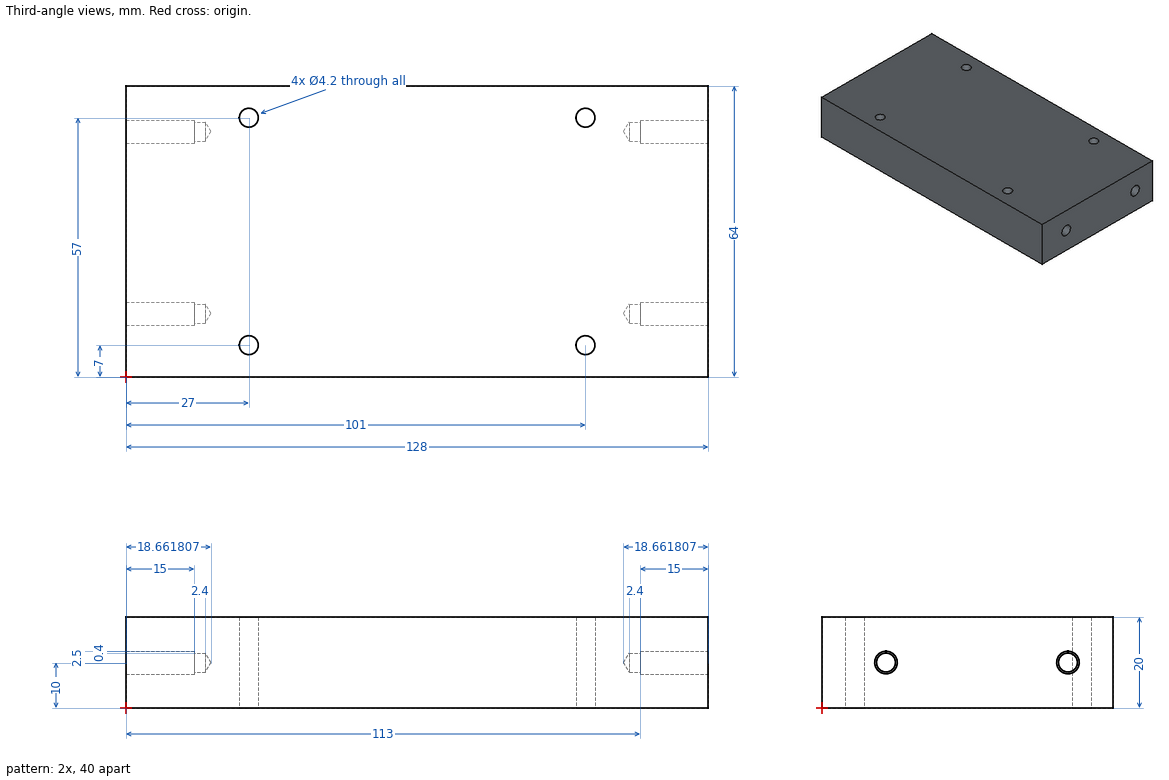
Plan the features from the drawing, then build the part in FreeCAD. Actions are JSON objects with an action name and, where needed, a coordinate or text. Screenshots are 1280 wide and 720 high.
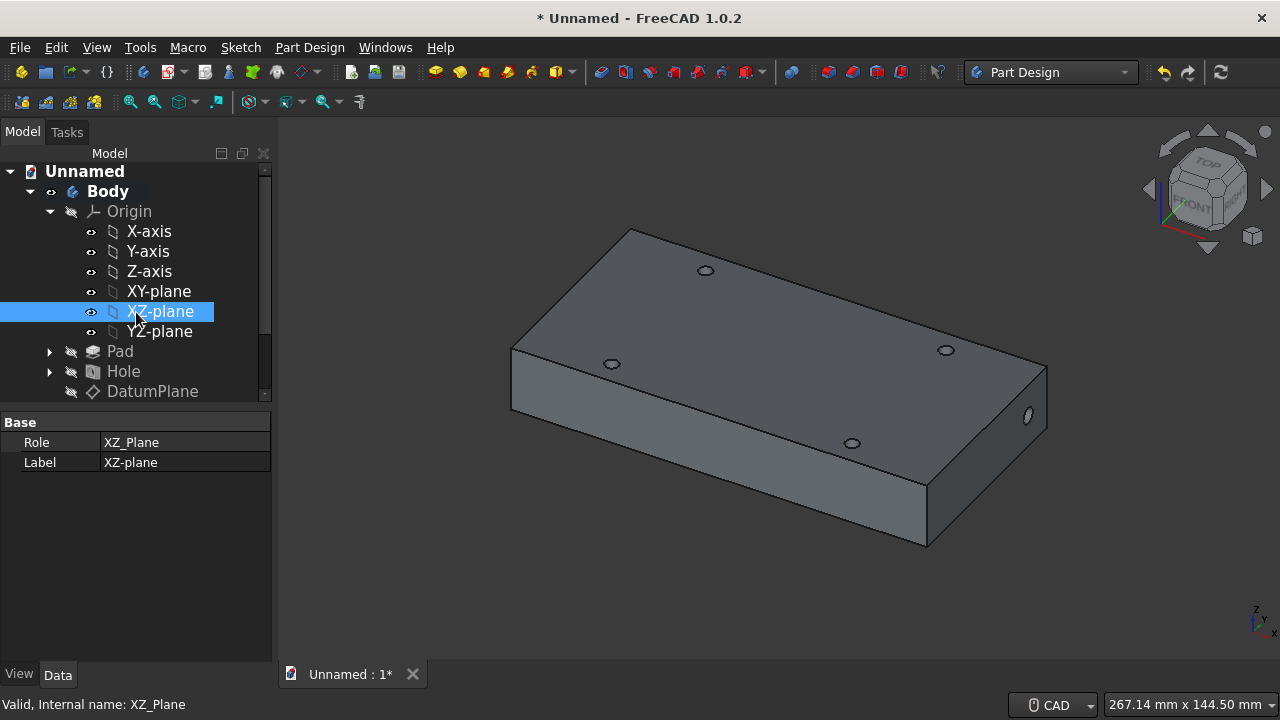
{"action": "left_click", "coordinate": [302, 72]}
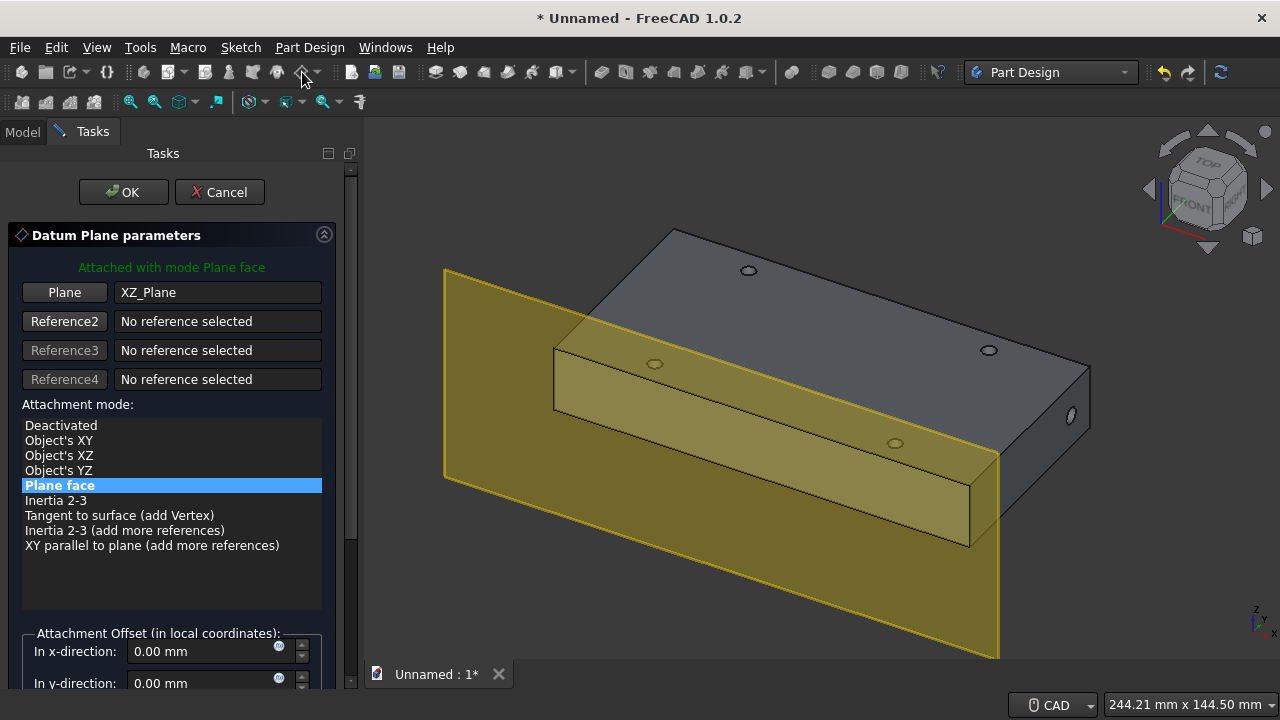
{"action": "scroll", "coordinate": [351, 426], "scroll_direction": "down", "scroll_amount": 2}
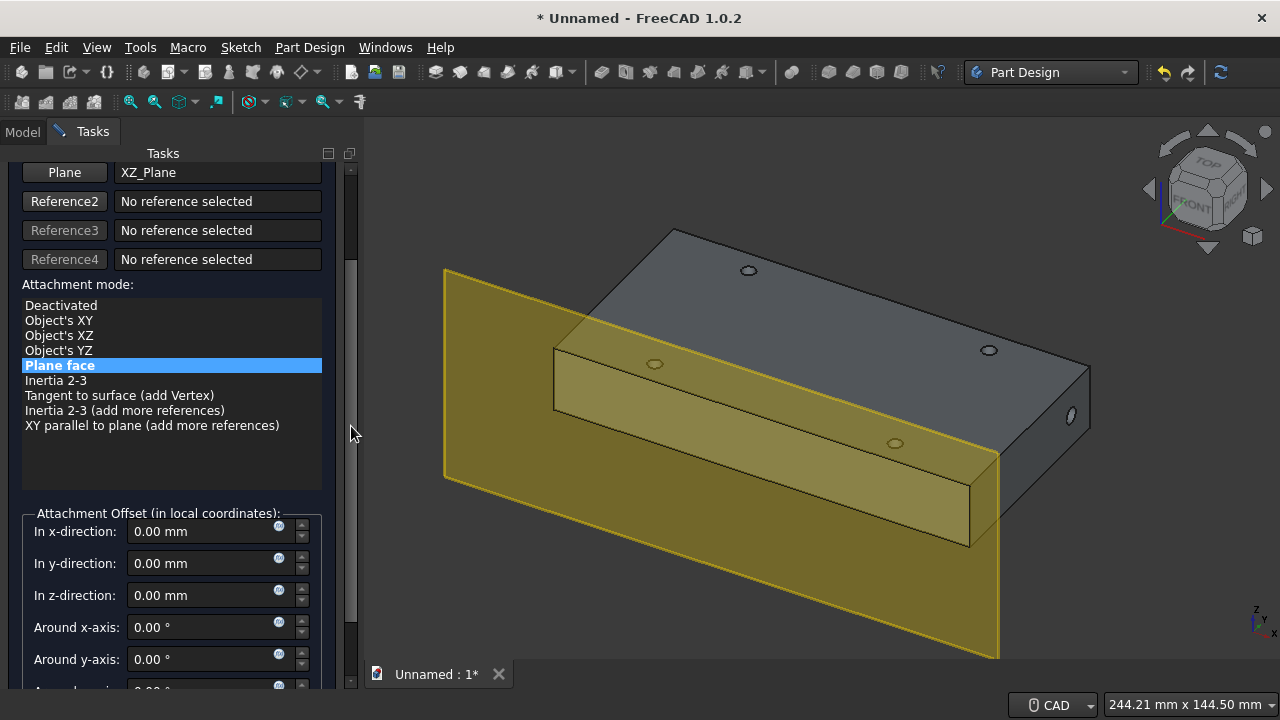
{"action": "triple_click", "coordinate": [210, 595]}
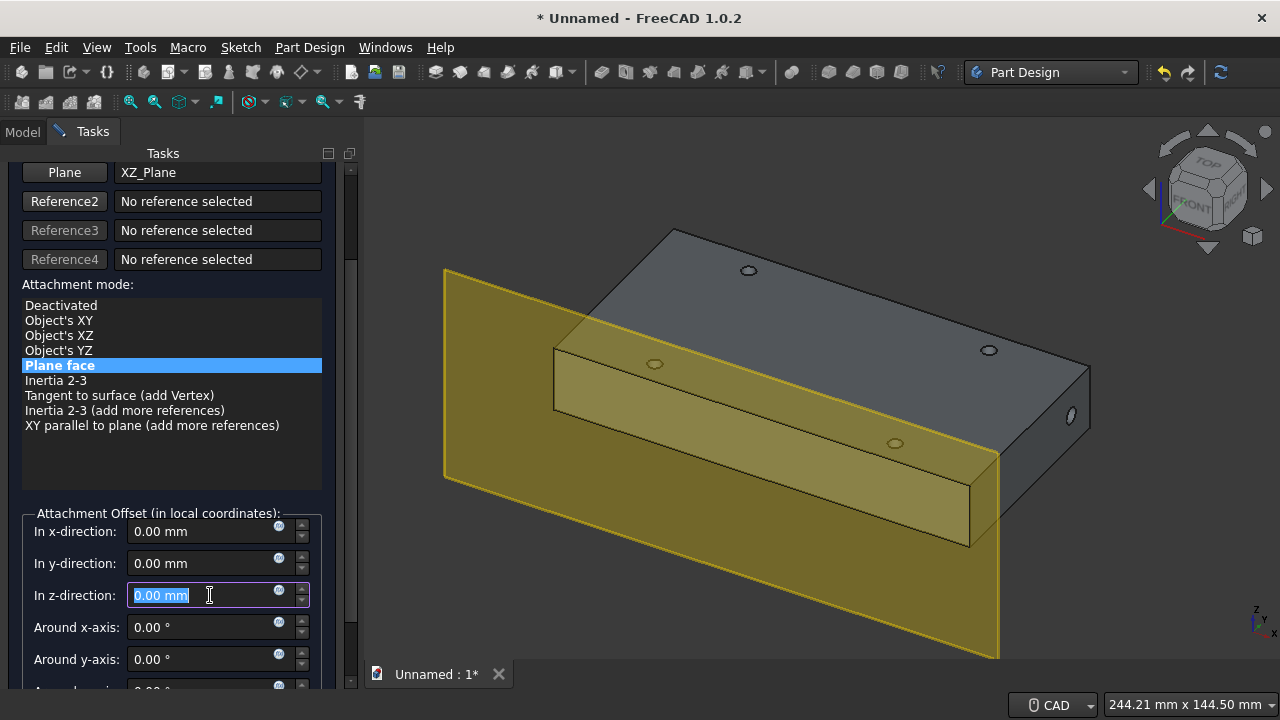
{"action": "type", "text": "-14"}
{"action": "key", "text": "Tab"}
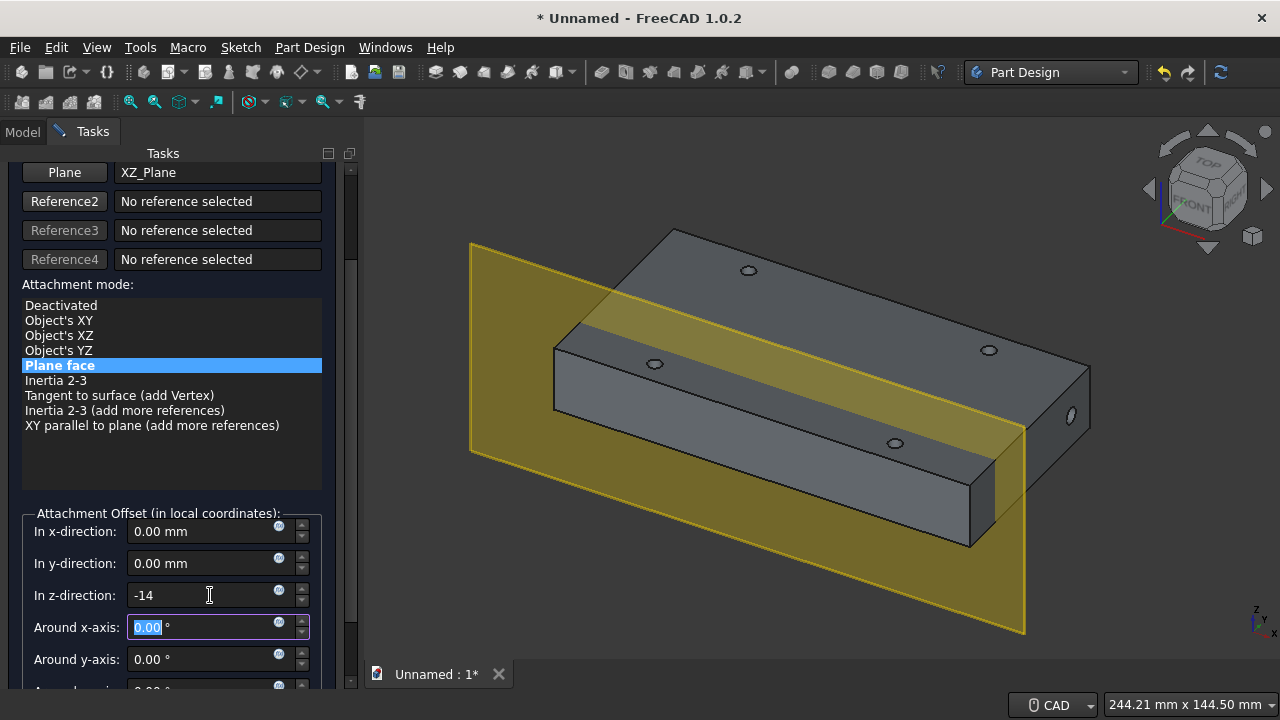
{"action": "scroll", "coordinate": [351, 426], "scroll_direction": "up", "scroll_amount": 3}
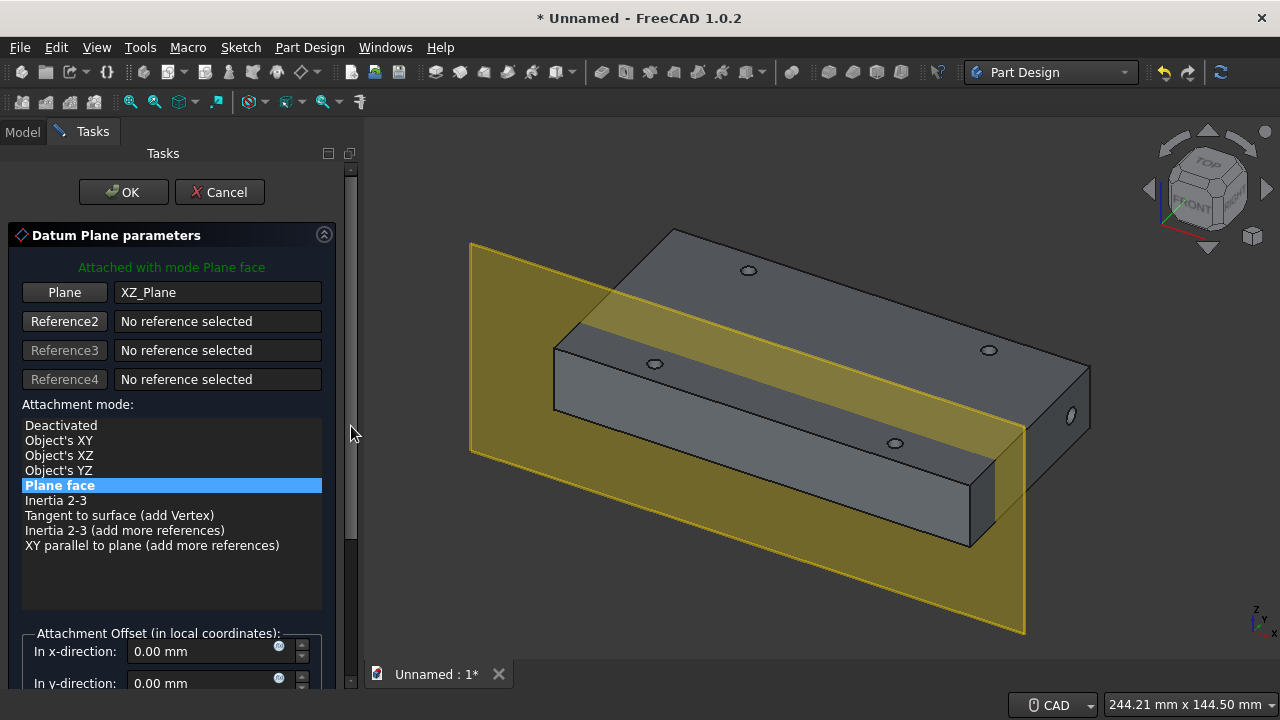
{"action": "left_click", "coordinate": [124, 192]}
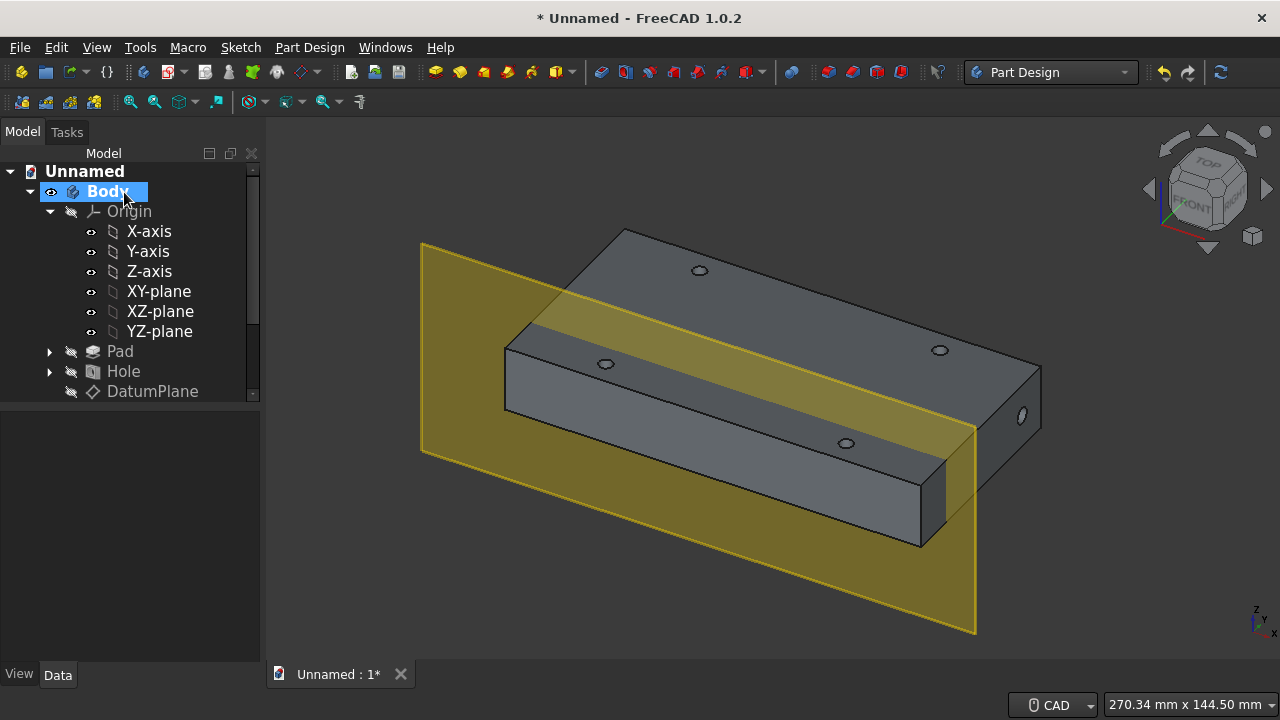
{"action": "scroll", "coordinate": [100, 287], "scroll_direction": "down", "scroll_amount": 3}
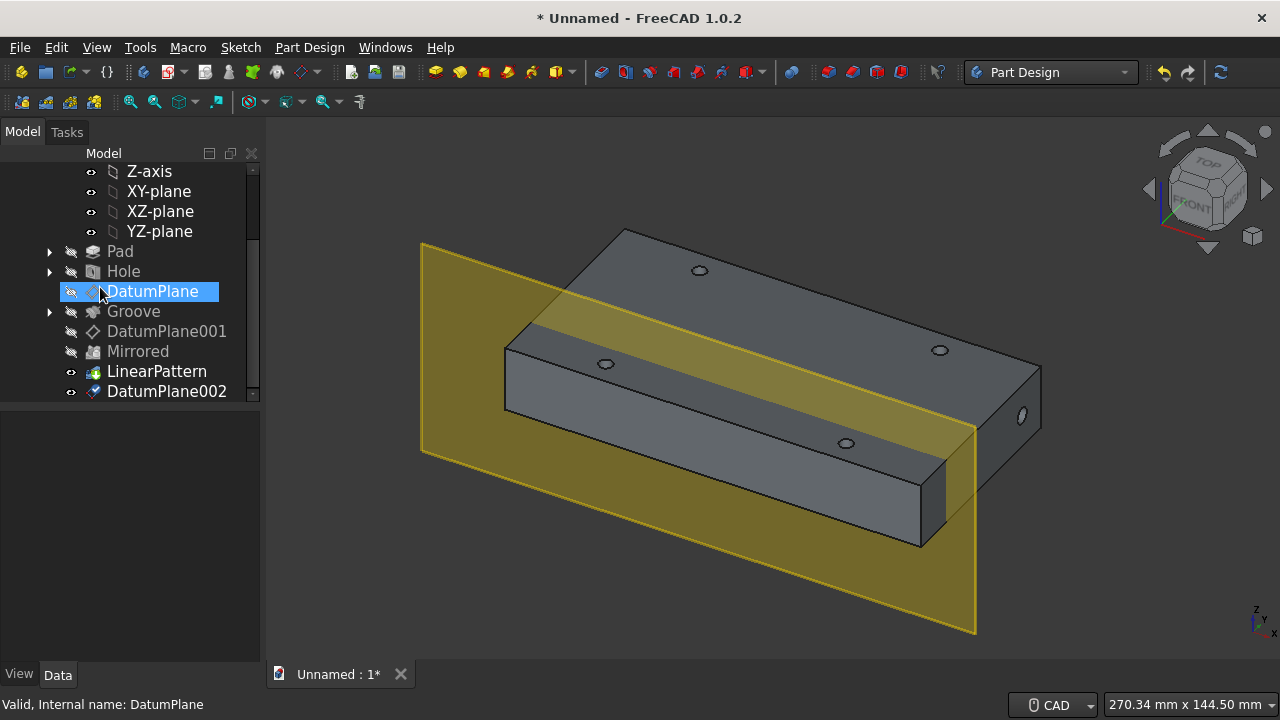
{"action": "left_click", "coordinate": [116, 392]}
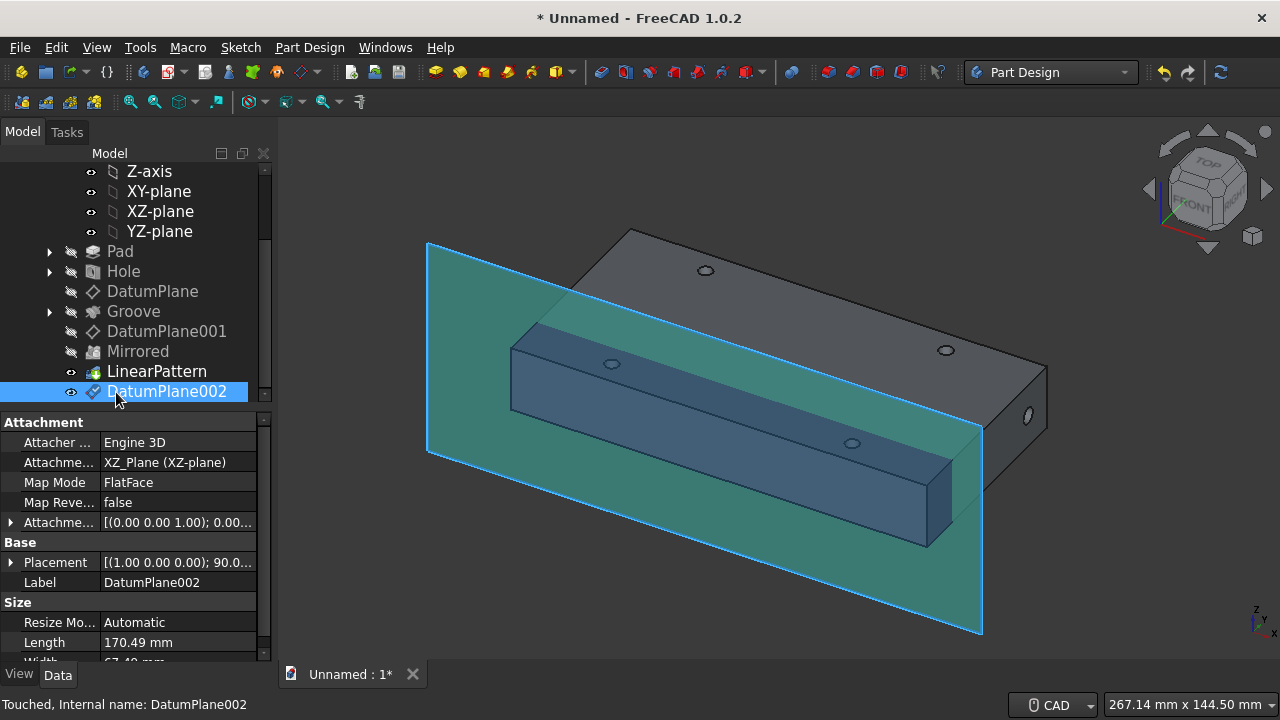
{"action": "left_click", "coordinate": [168, 72]}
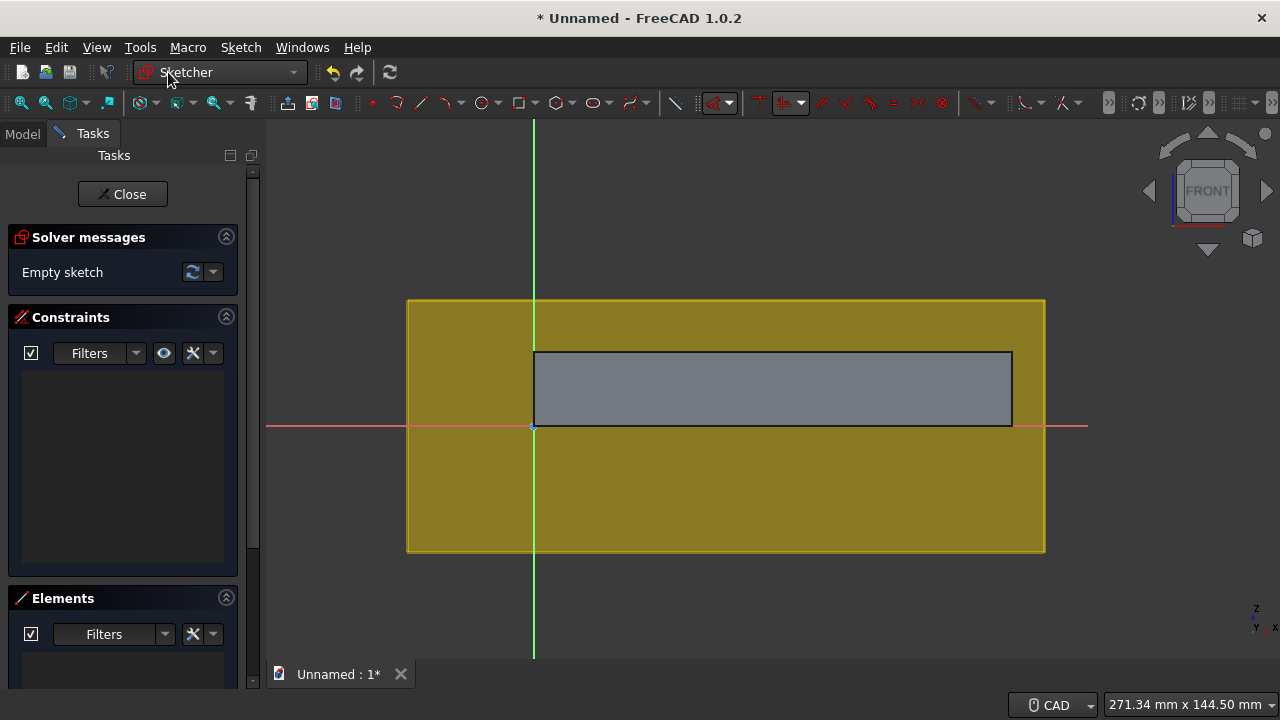
{"action": "left_click", "coordinate": [336, 104]}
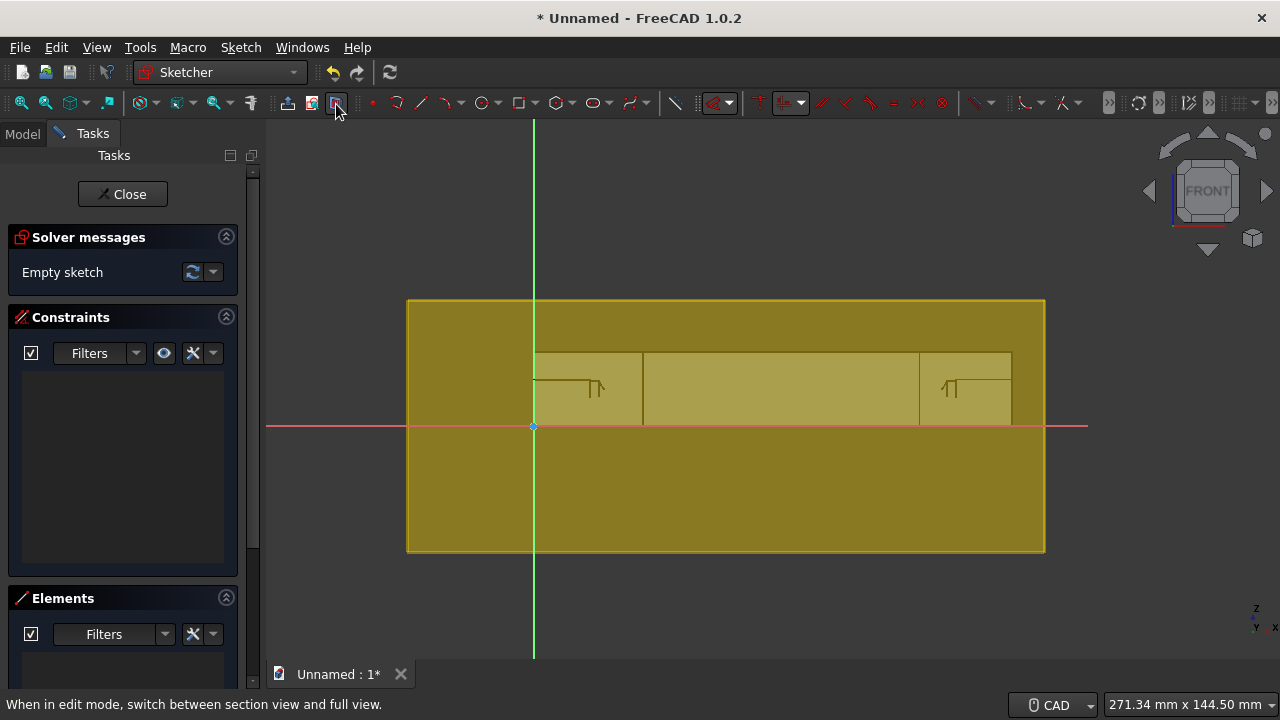
{"action": "scroll", "coordinate": [1048, 383], "scroll_direction": "up", "scroll_amount": 9}